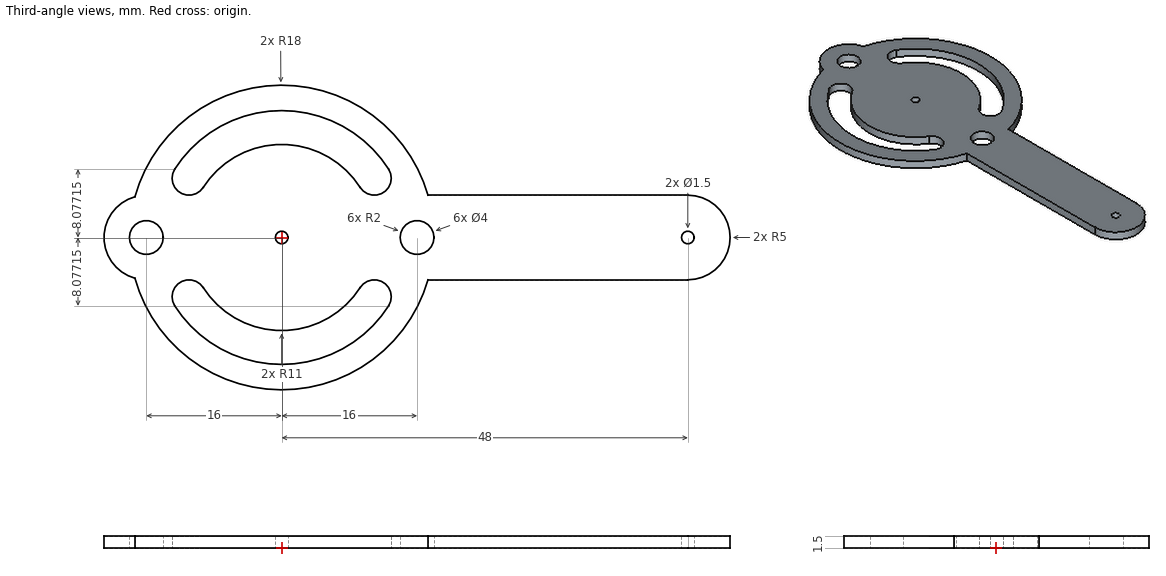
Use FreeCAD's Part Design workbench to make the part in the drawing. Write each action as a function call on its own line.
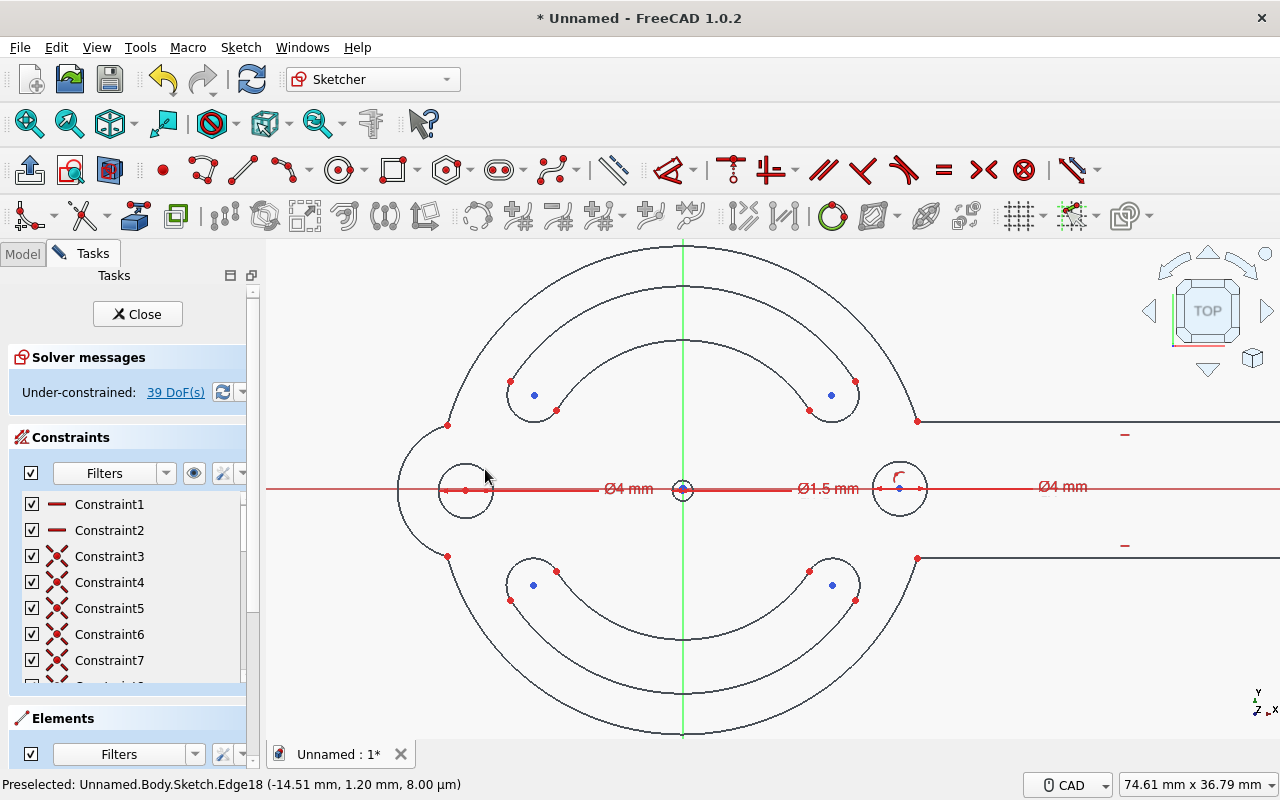
click(1042, 558)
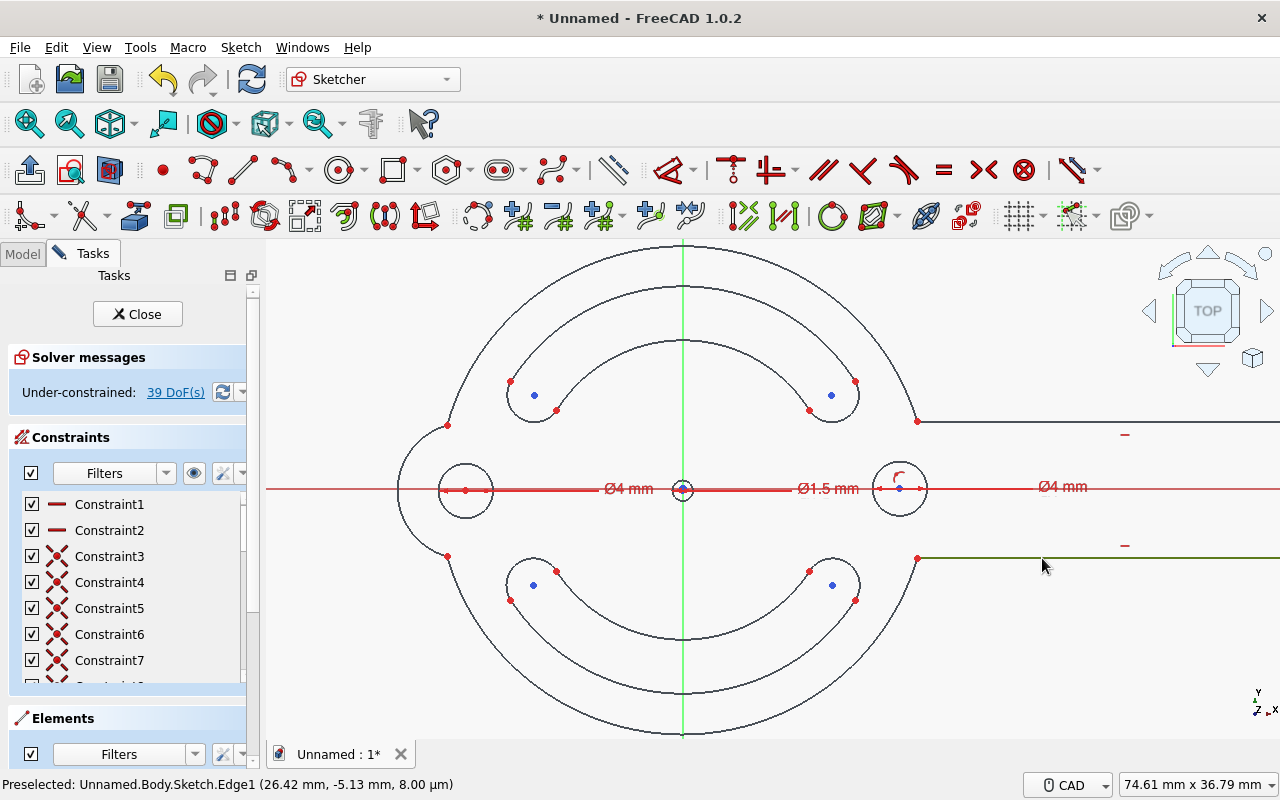
scroll(466, 489, down, 3)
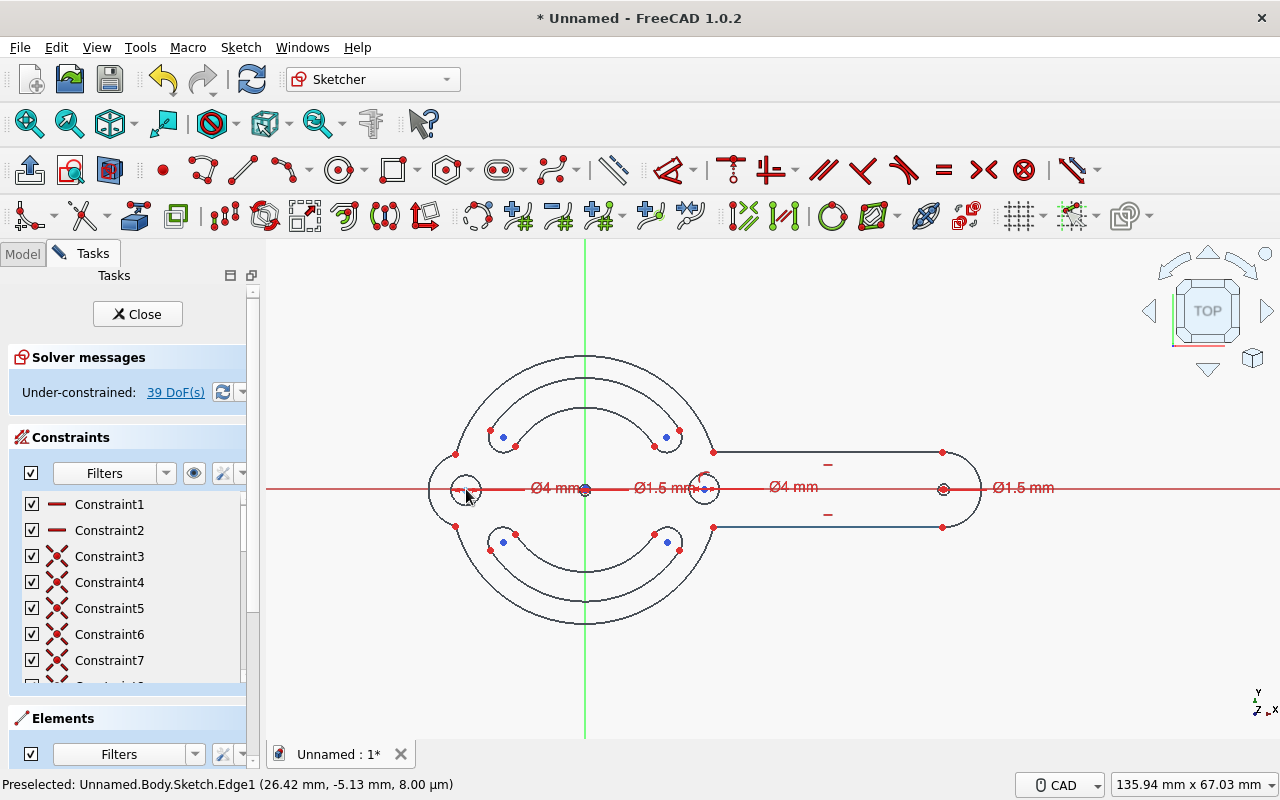
click(974, 512)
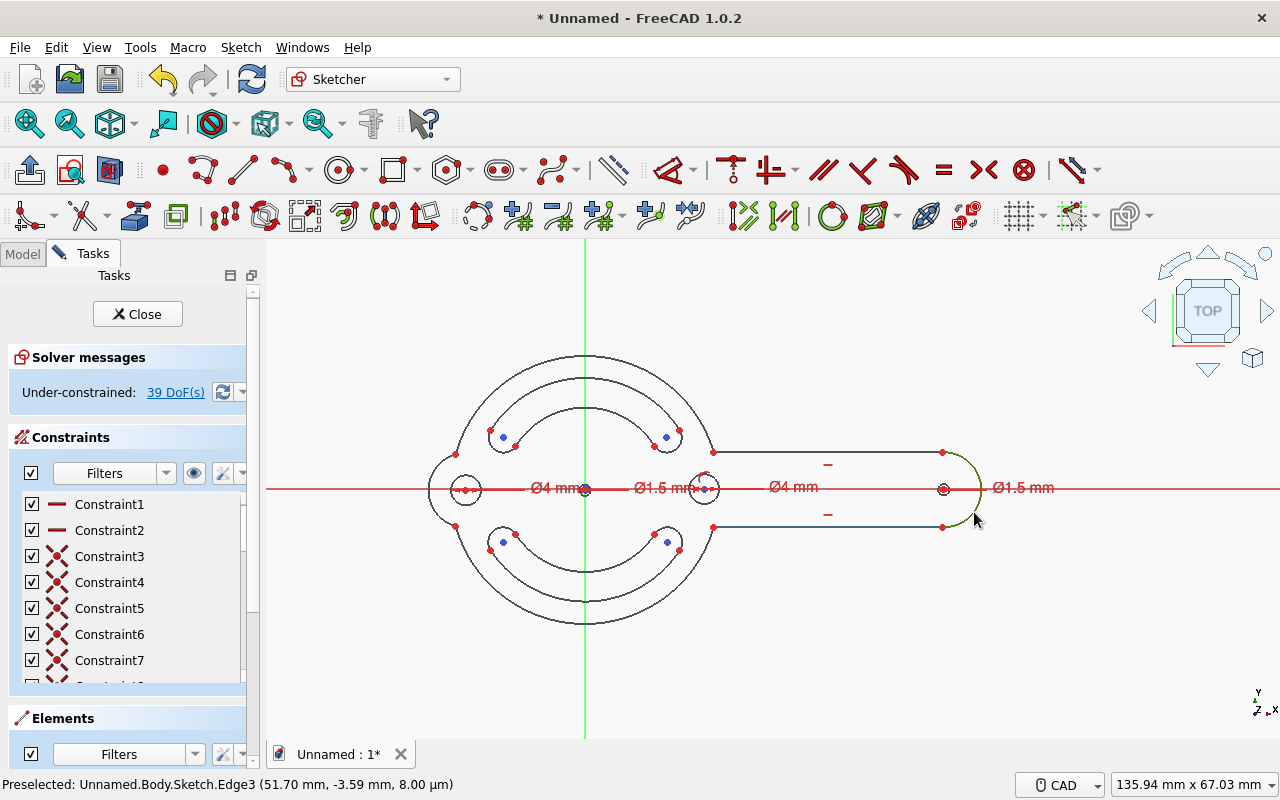
click(904, 170)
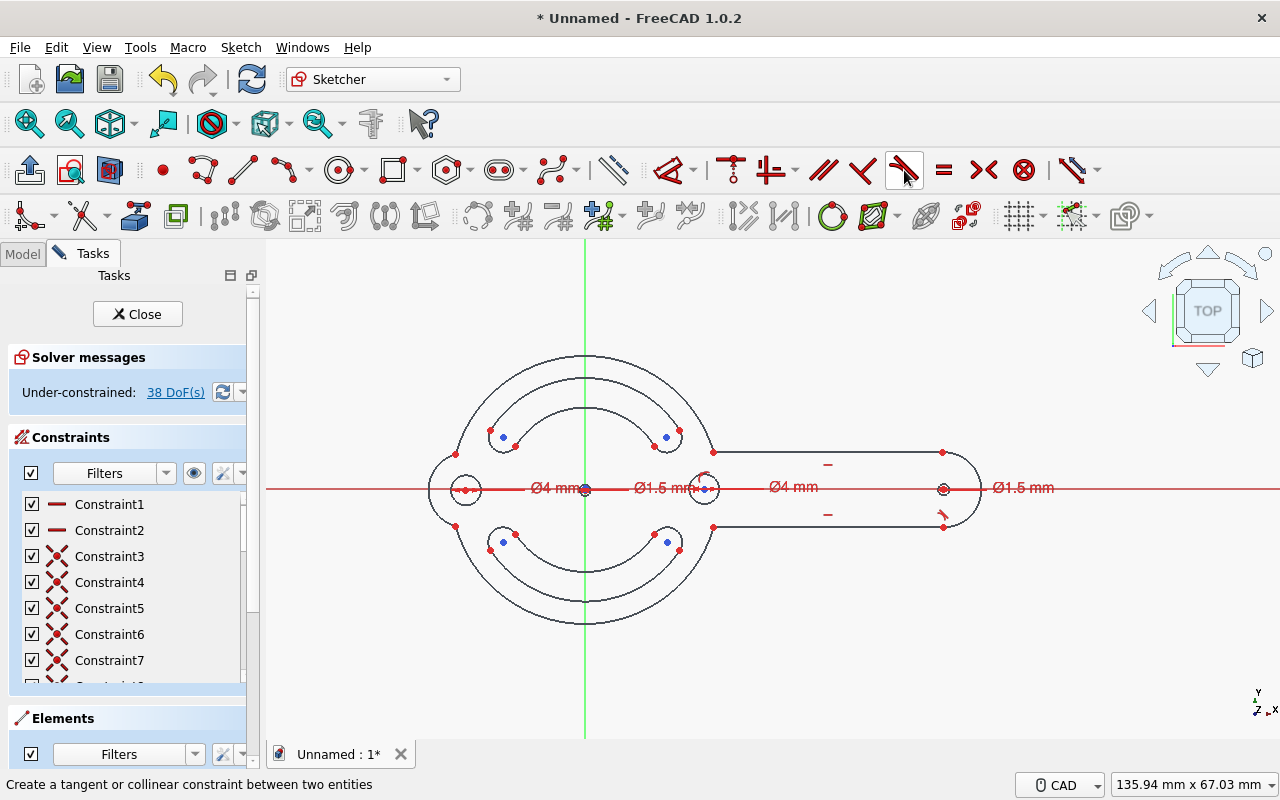
click(874, 452)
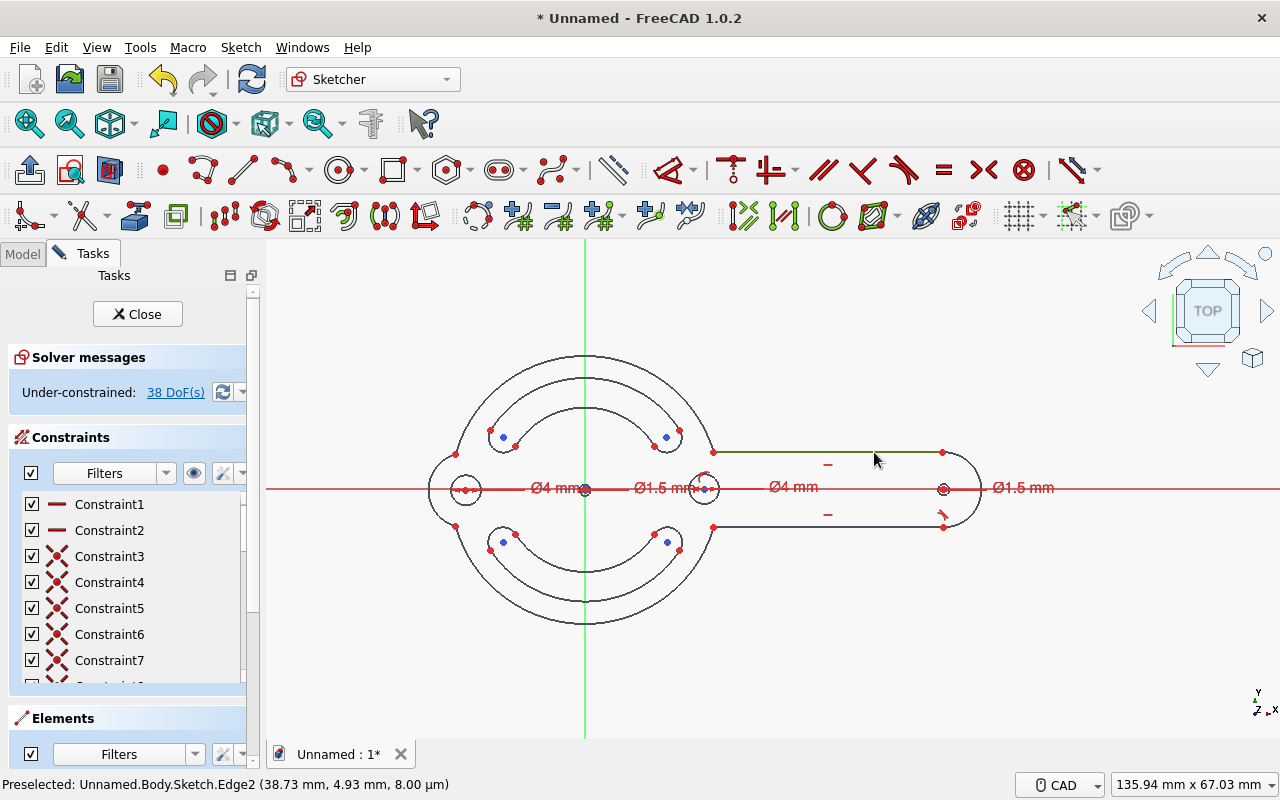
click(974, 512)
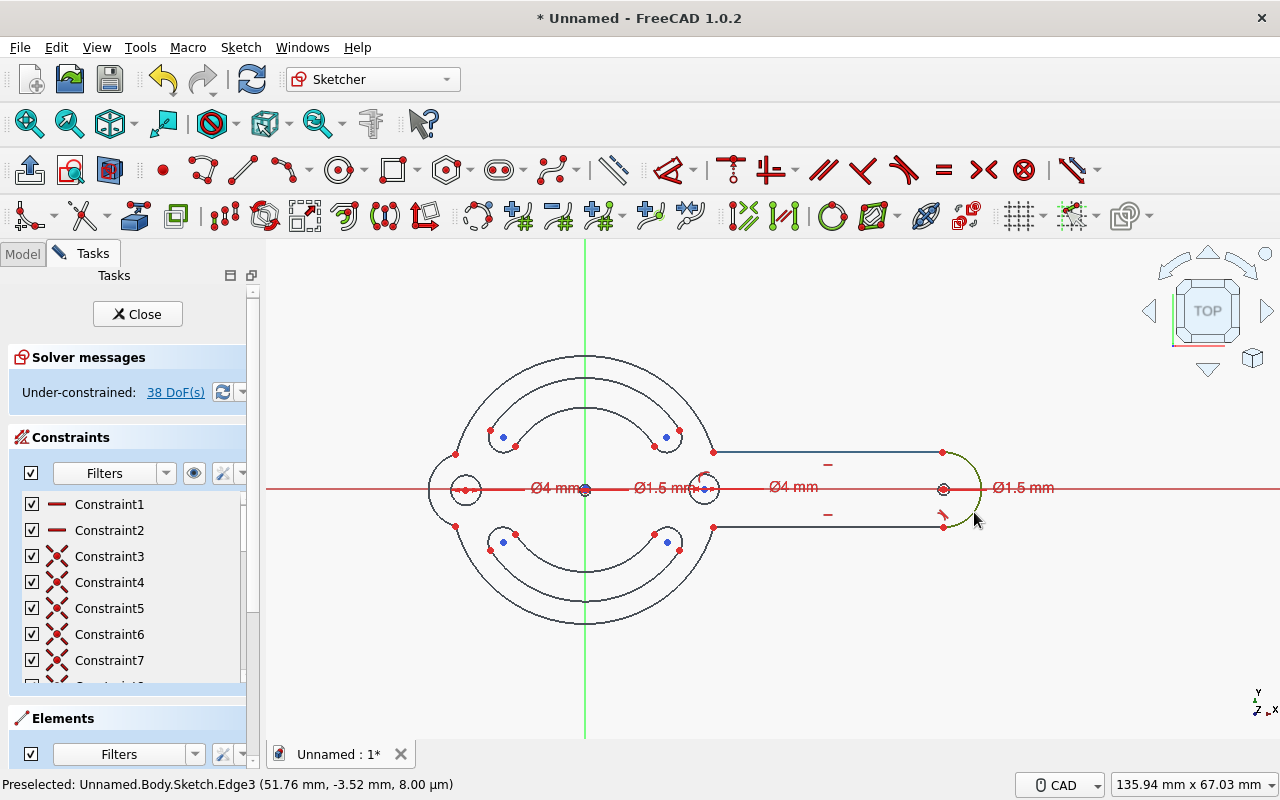
click(904, 170)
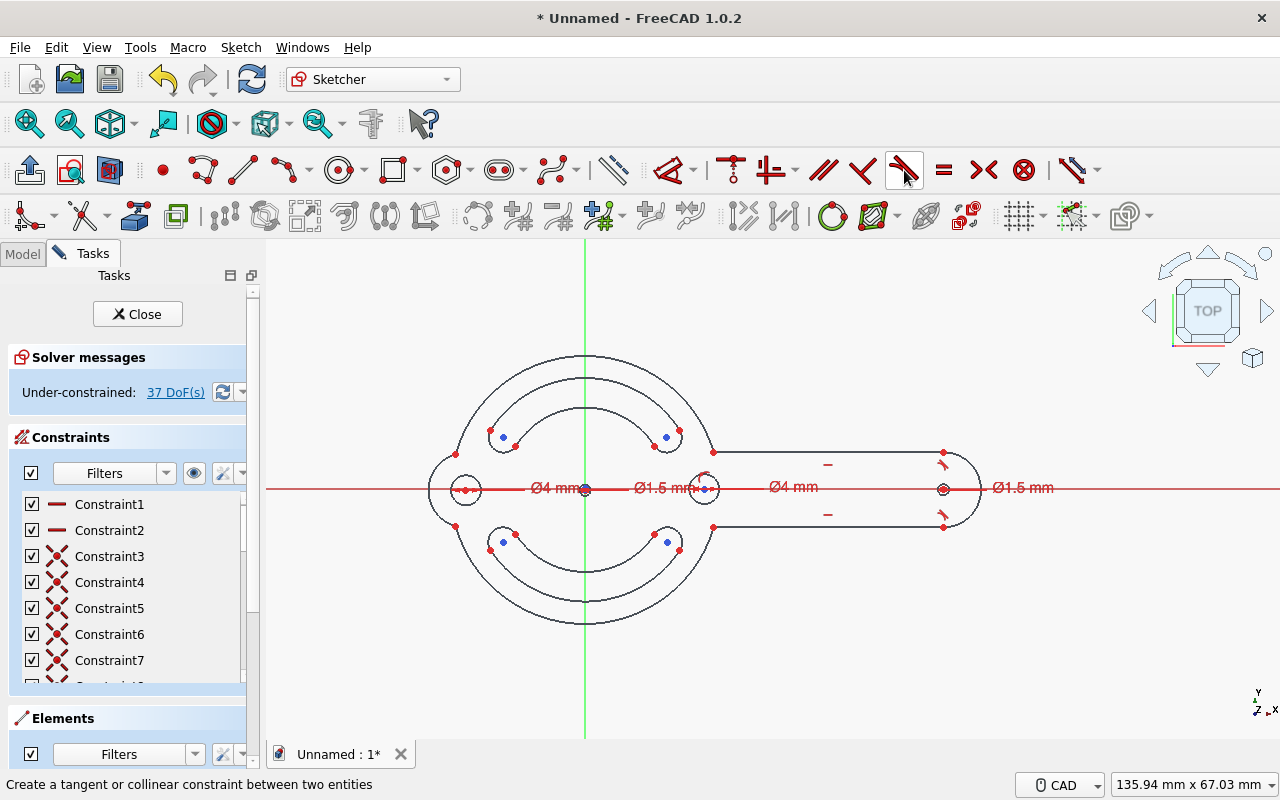
click(553, 565)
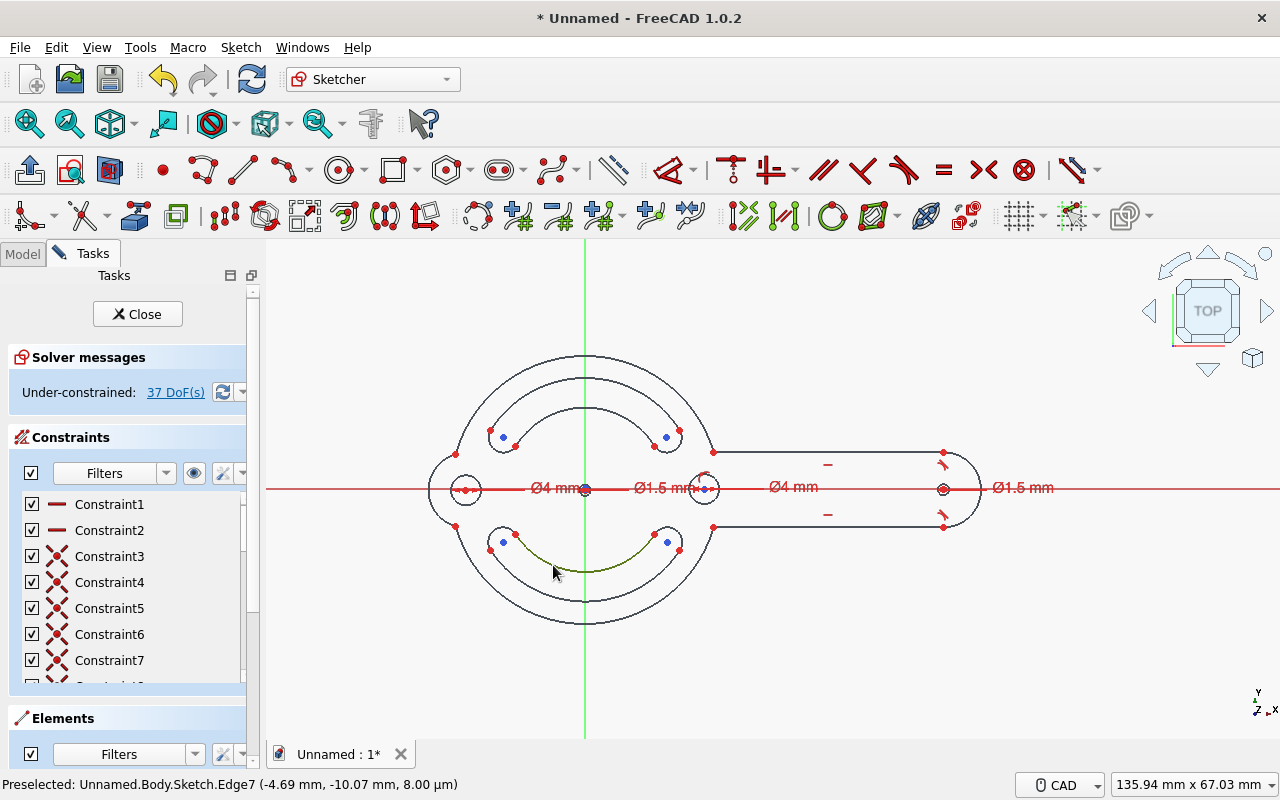
click(681, 537)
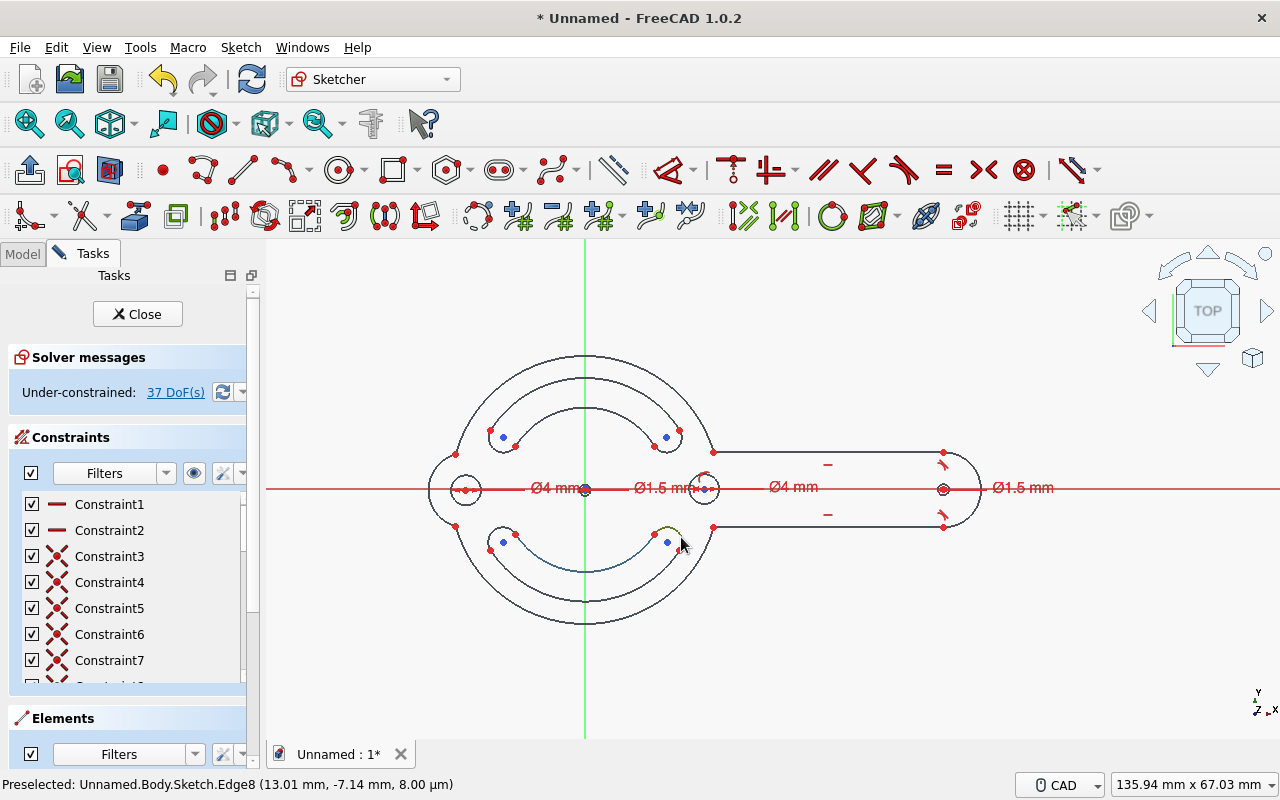
click(904, 170)